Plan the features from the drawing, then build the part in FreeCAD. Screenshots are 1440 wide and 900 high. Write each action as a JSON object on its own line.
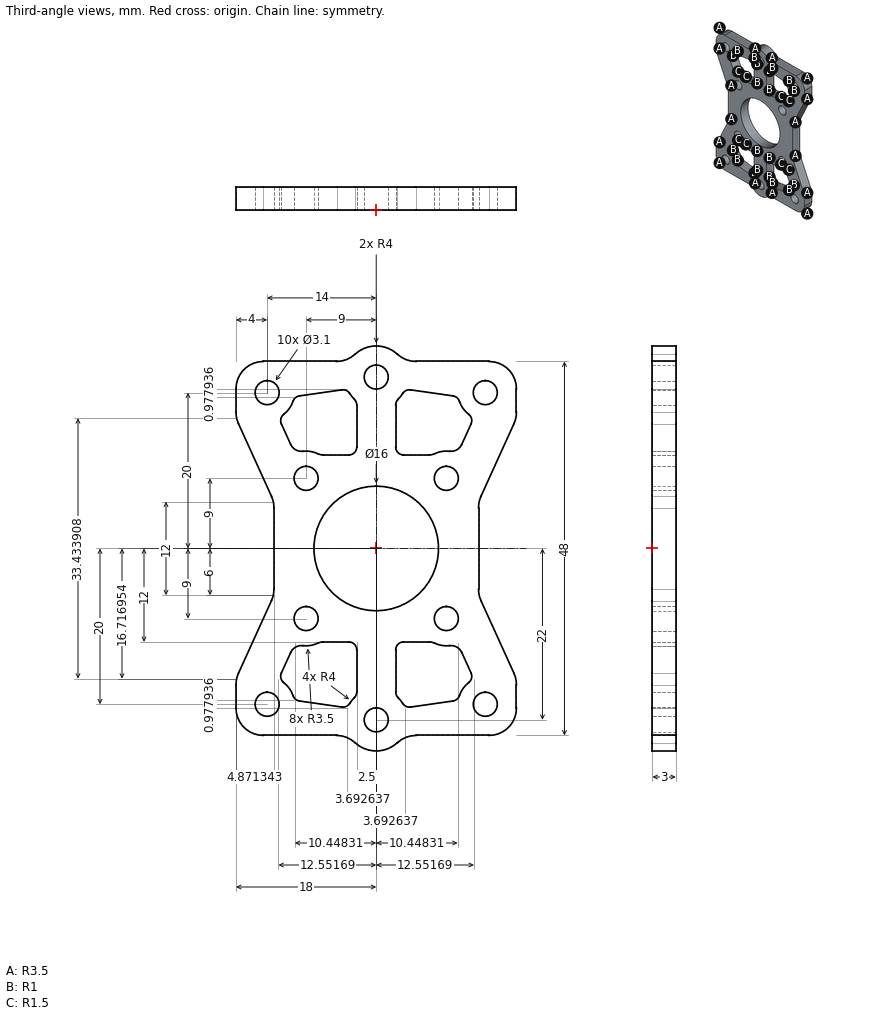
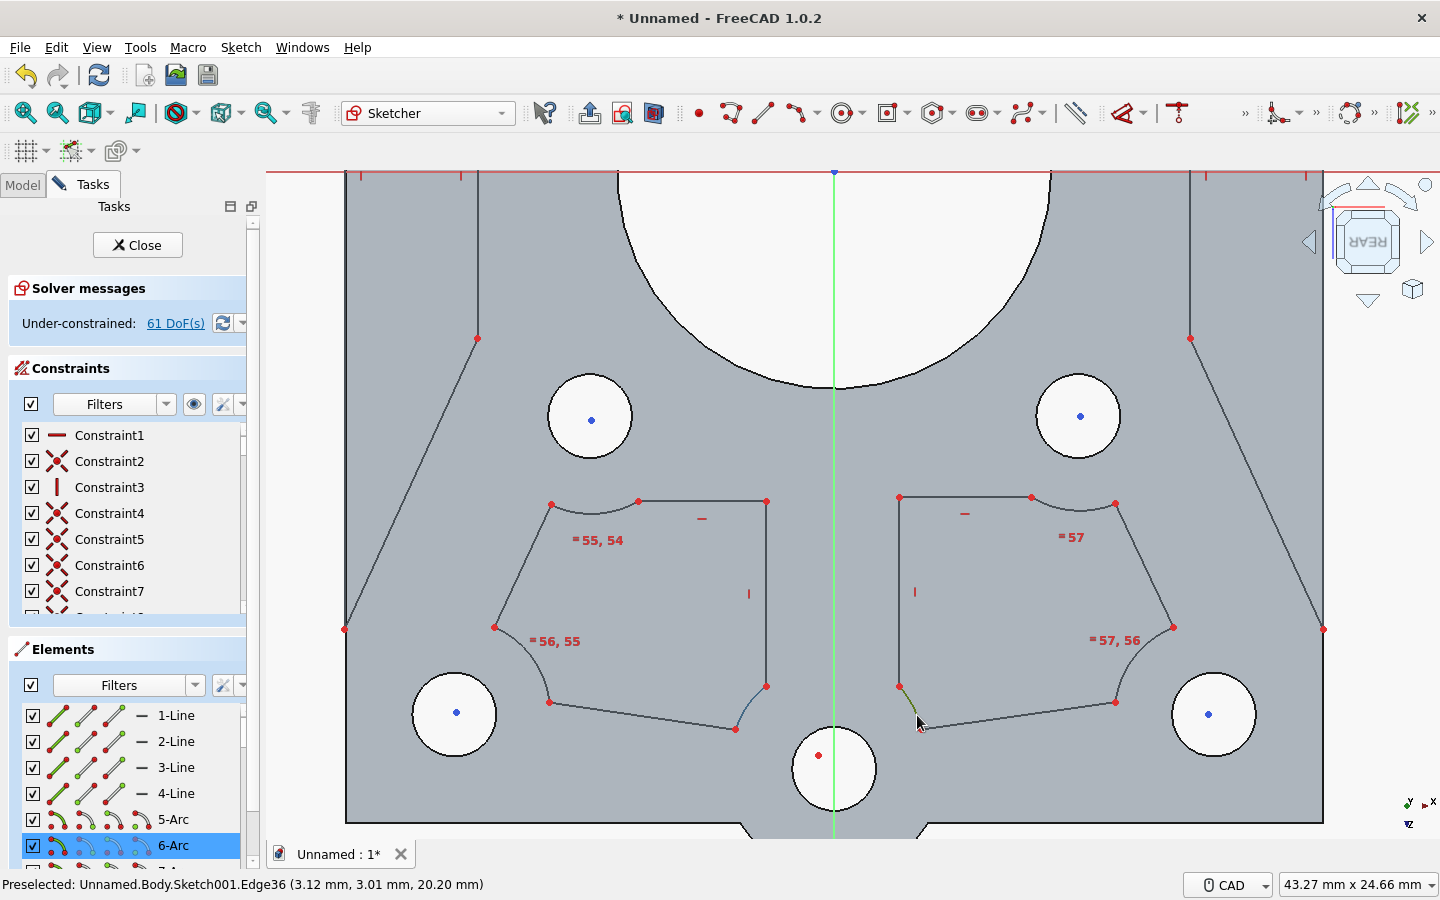
{"action": "key", "text": "e"}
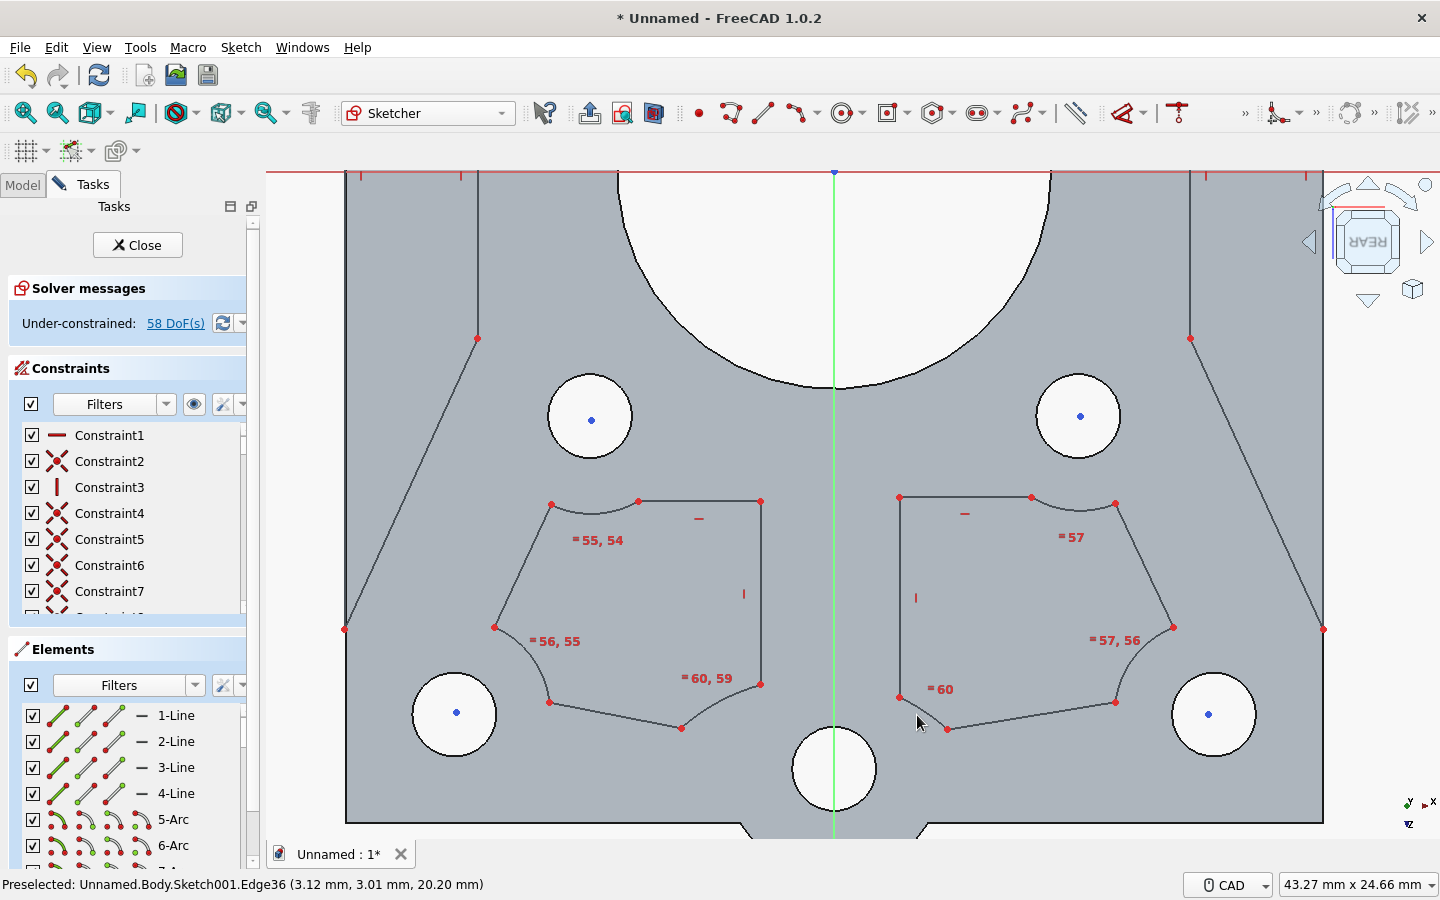
{"action": "scroll", "coordinate": [756, 698], "scroll_direction": "down", "scroll_amount": 5}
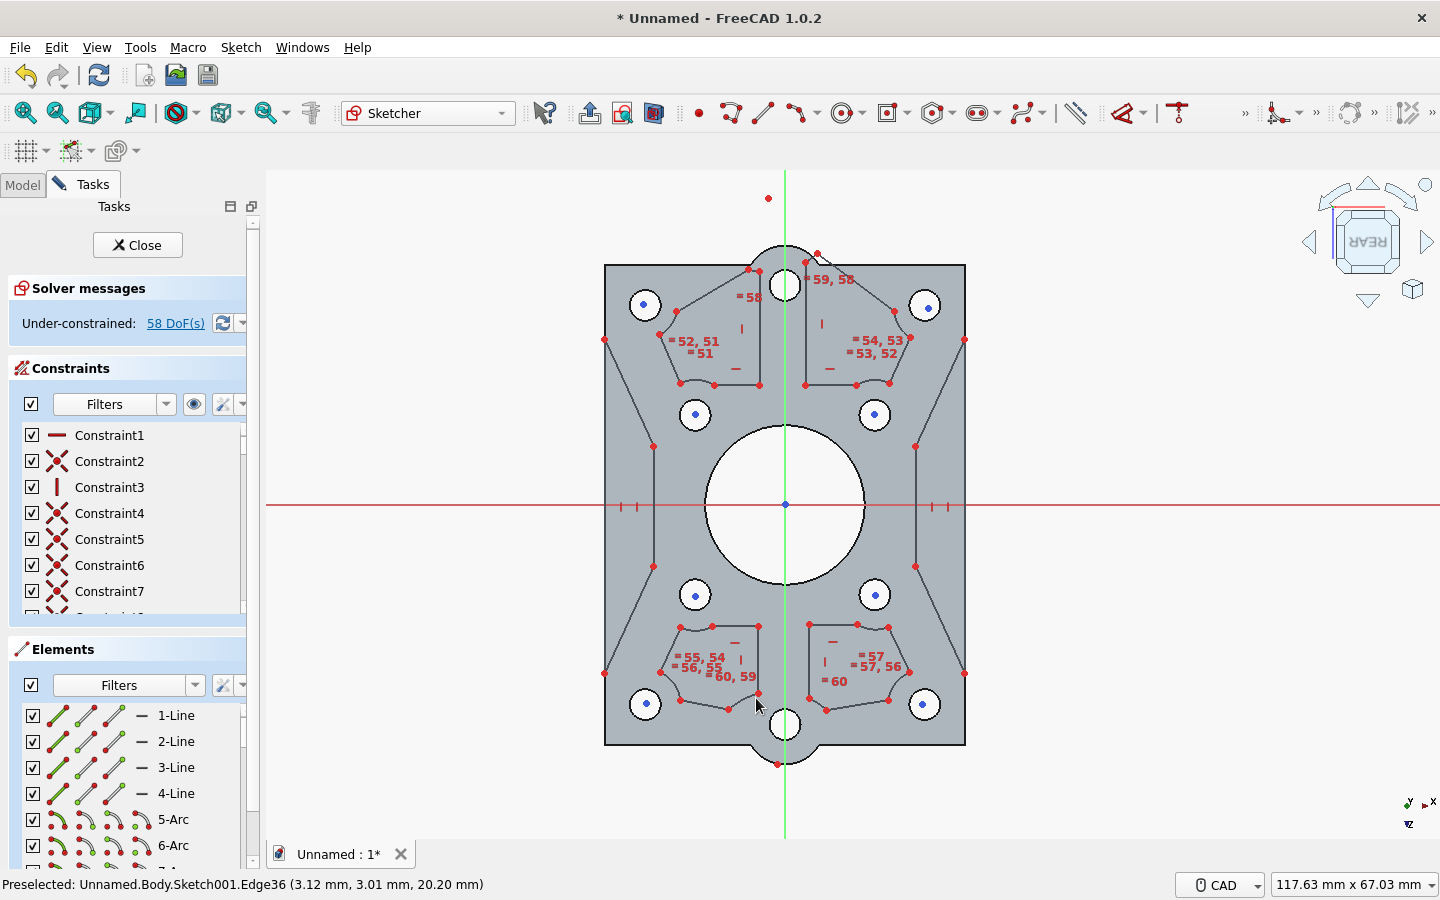
{"action": "left_click", "coordinate": [768, 199]}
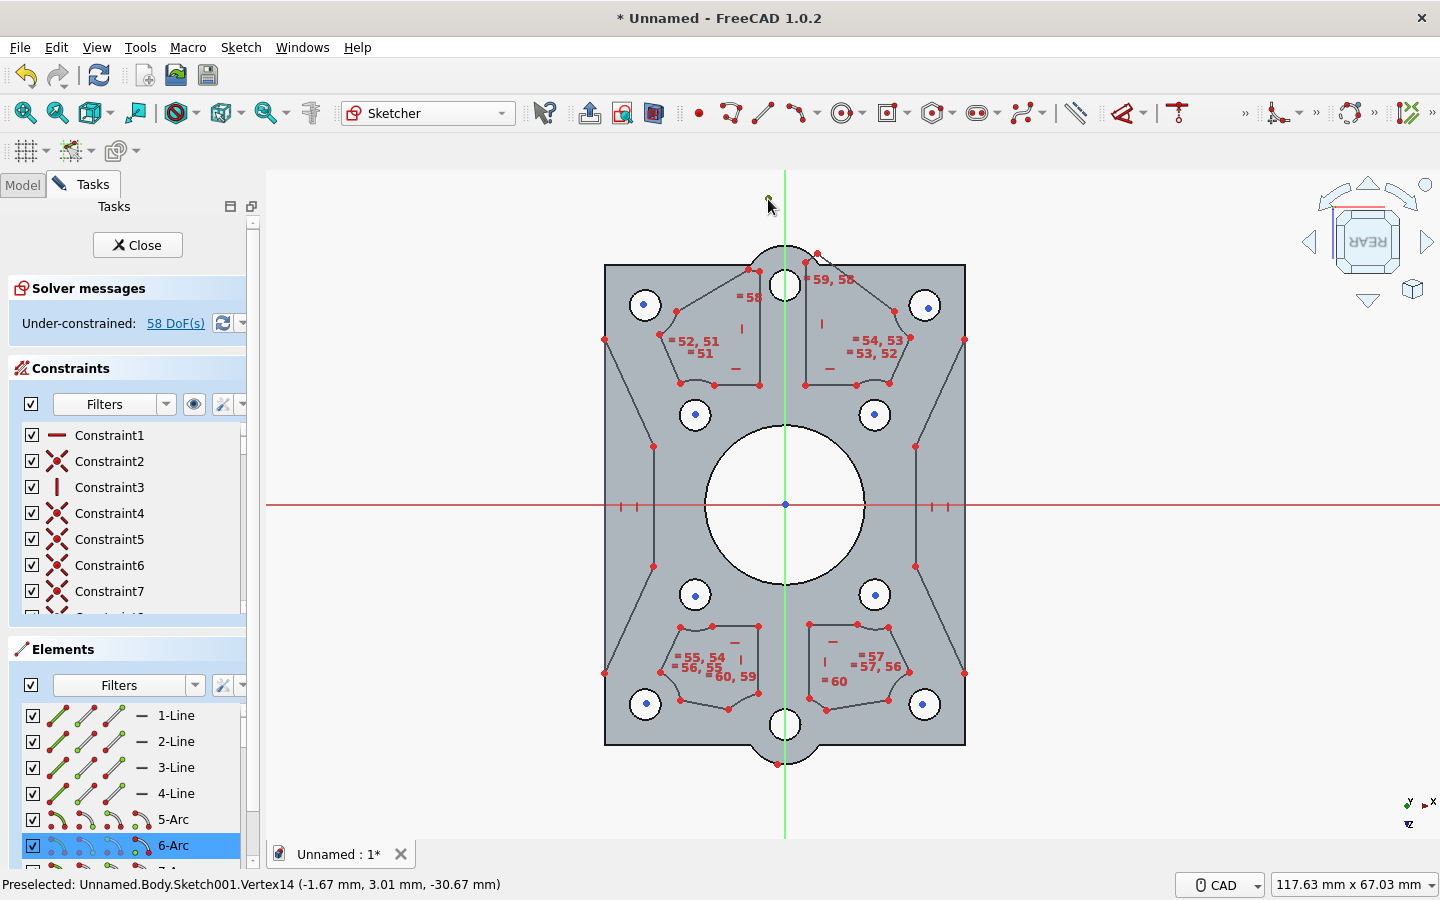
{"action": "left_click", "coordinate": [785, 767]}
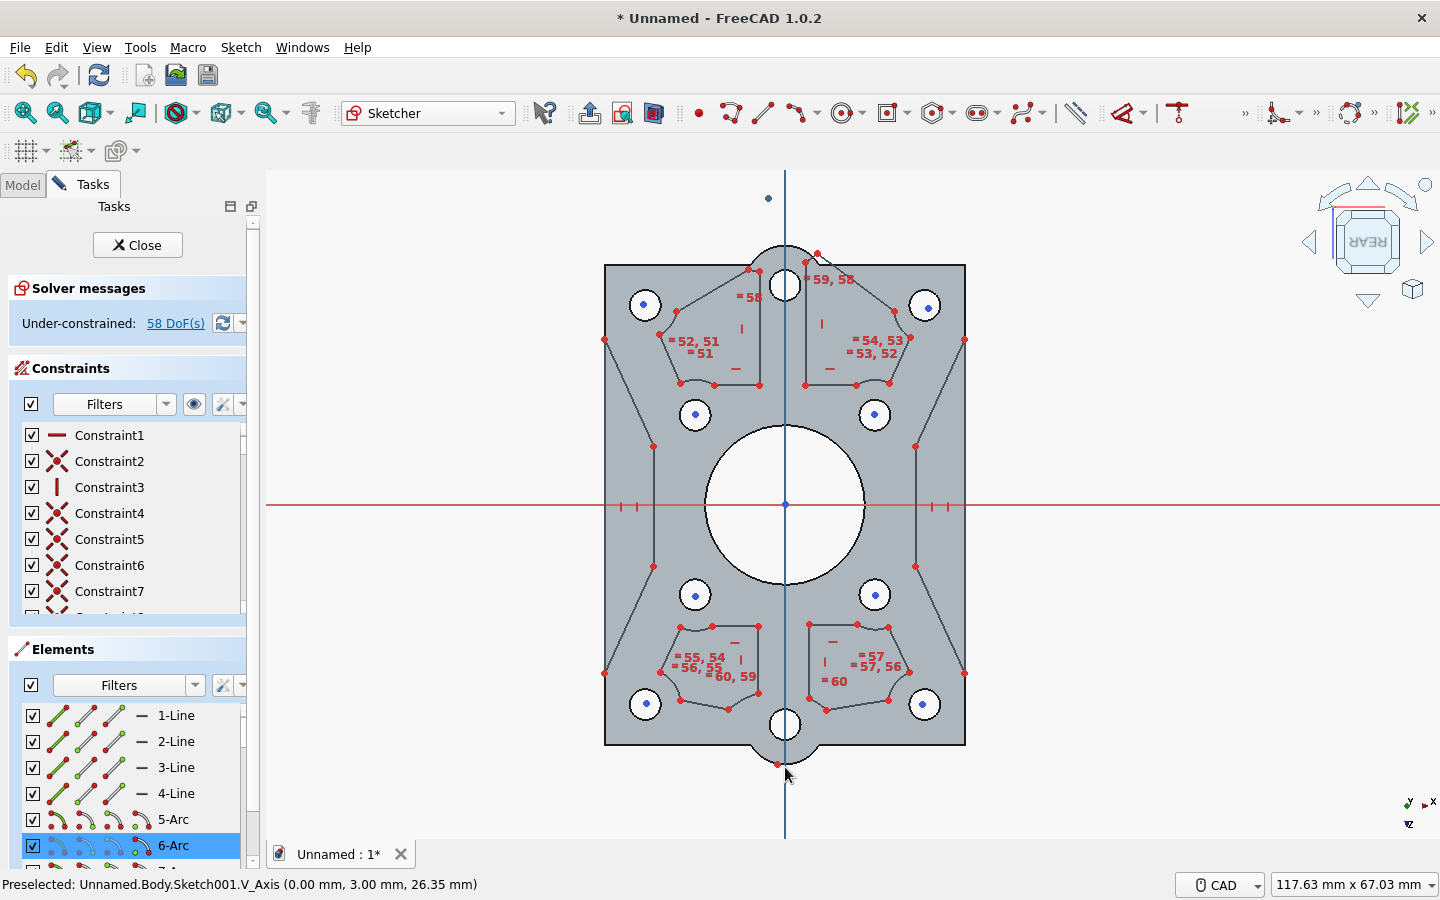
{"action": "key", "text": "c"}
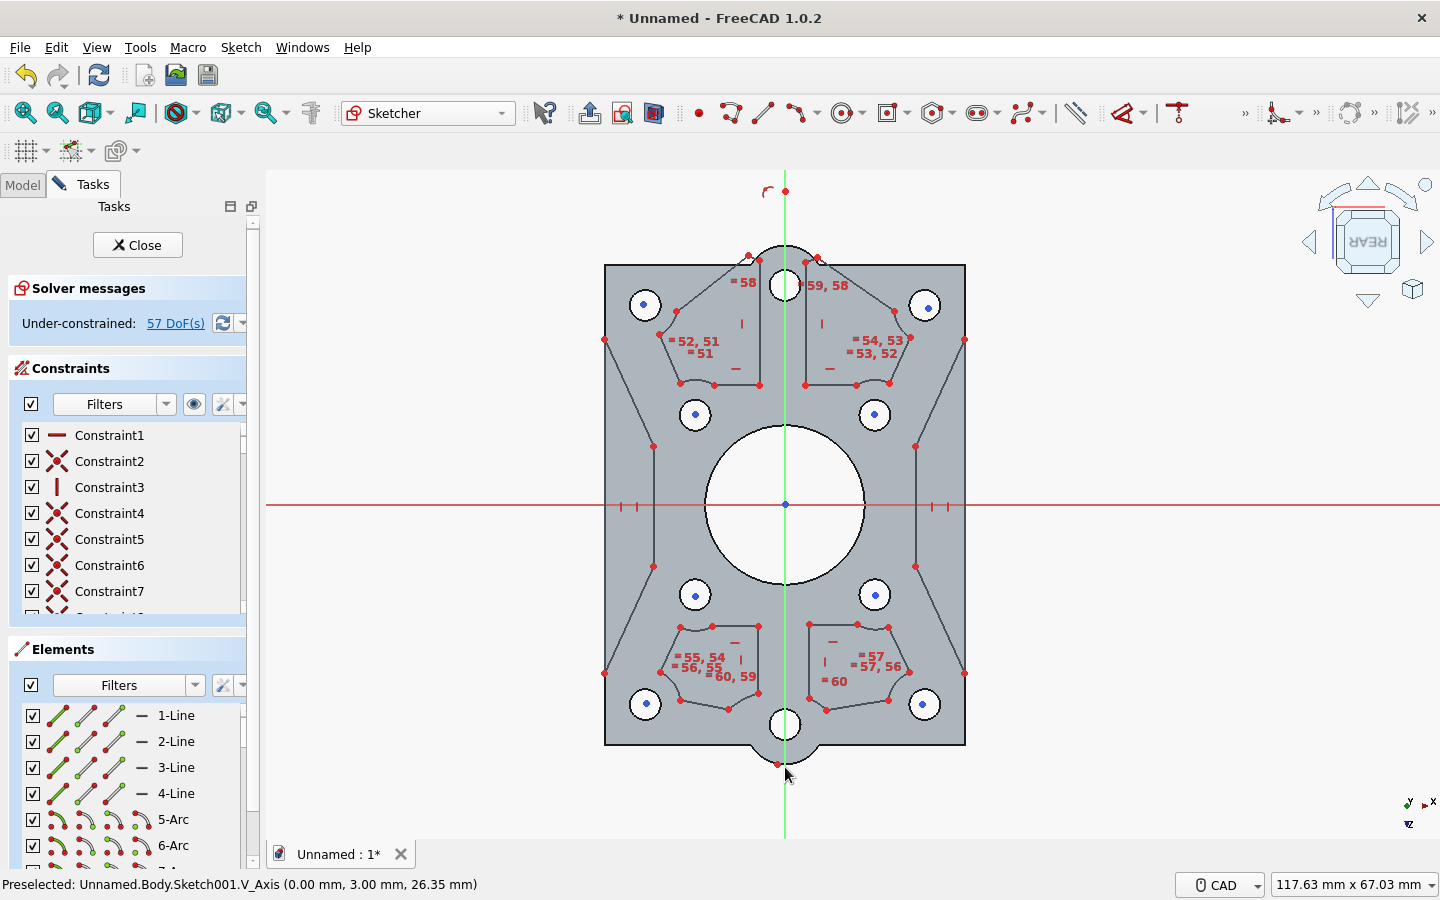
{"action": "left_click", "coordinate": [777, 765]}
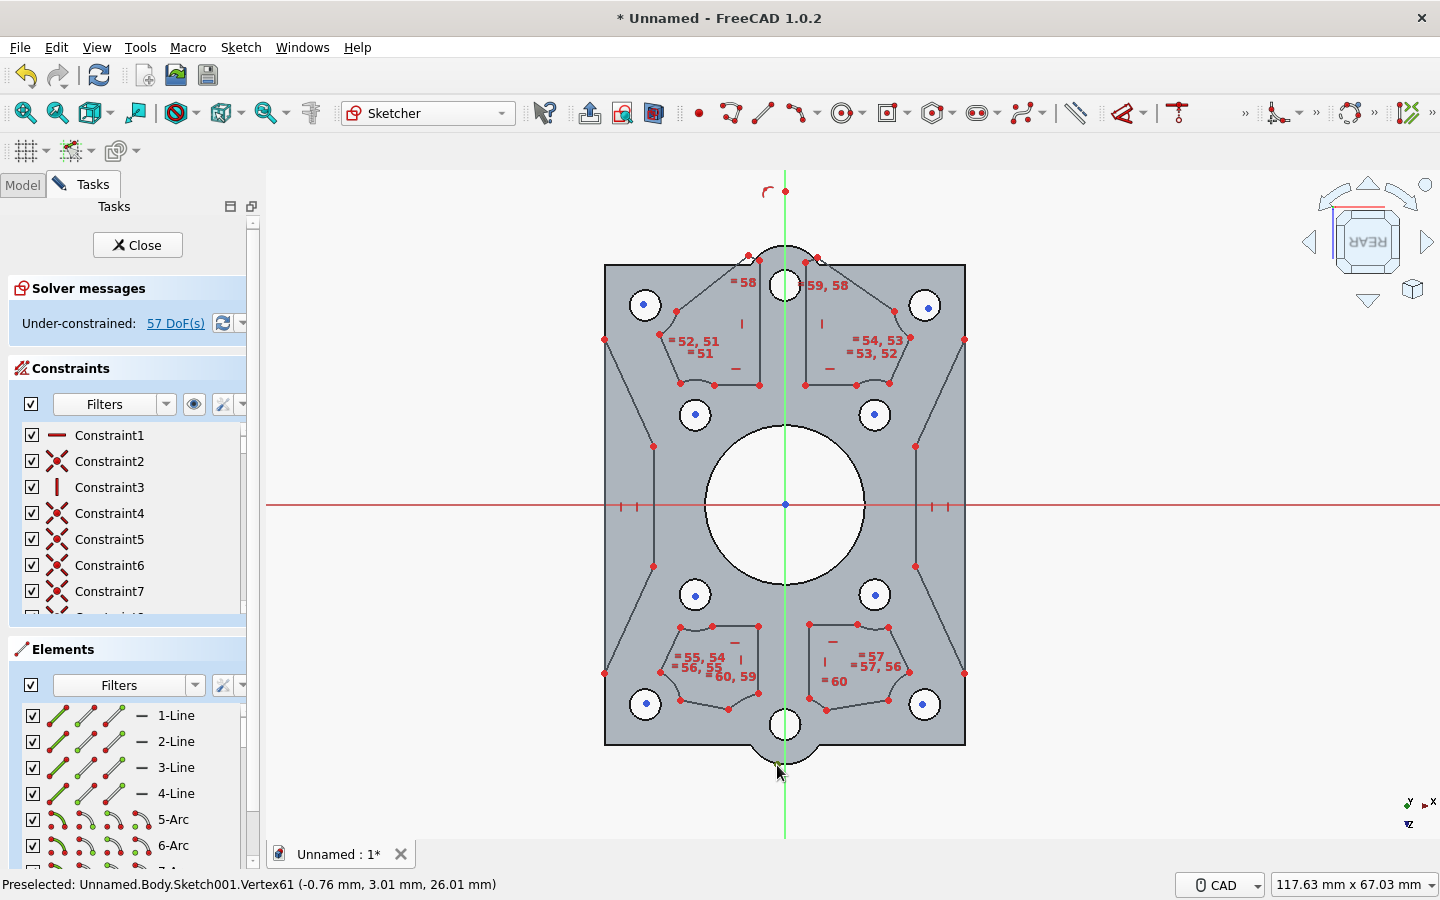
{"action": "left_click", "coordinate": [785, 767]}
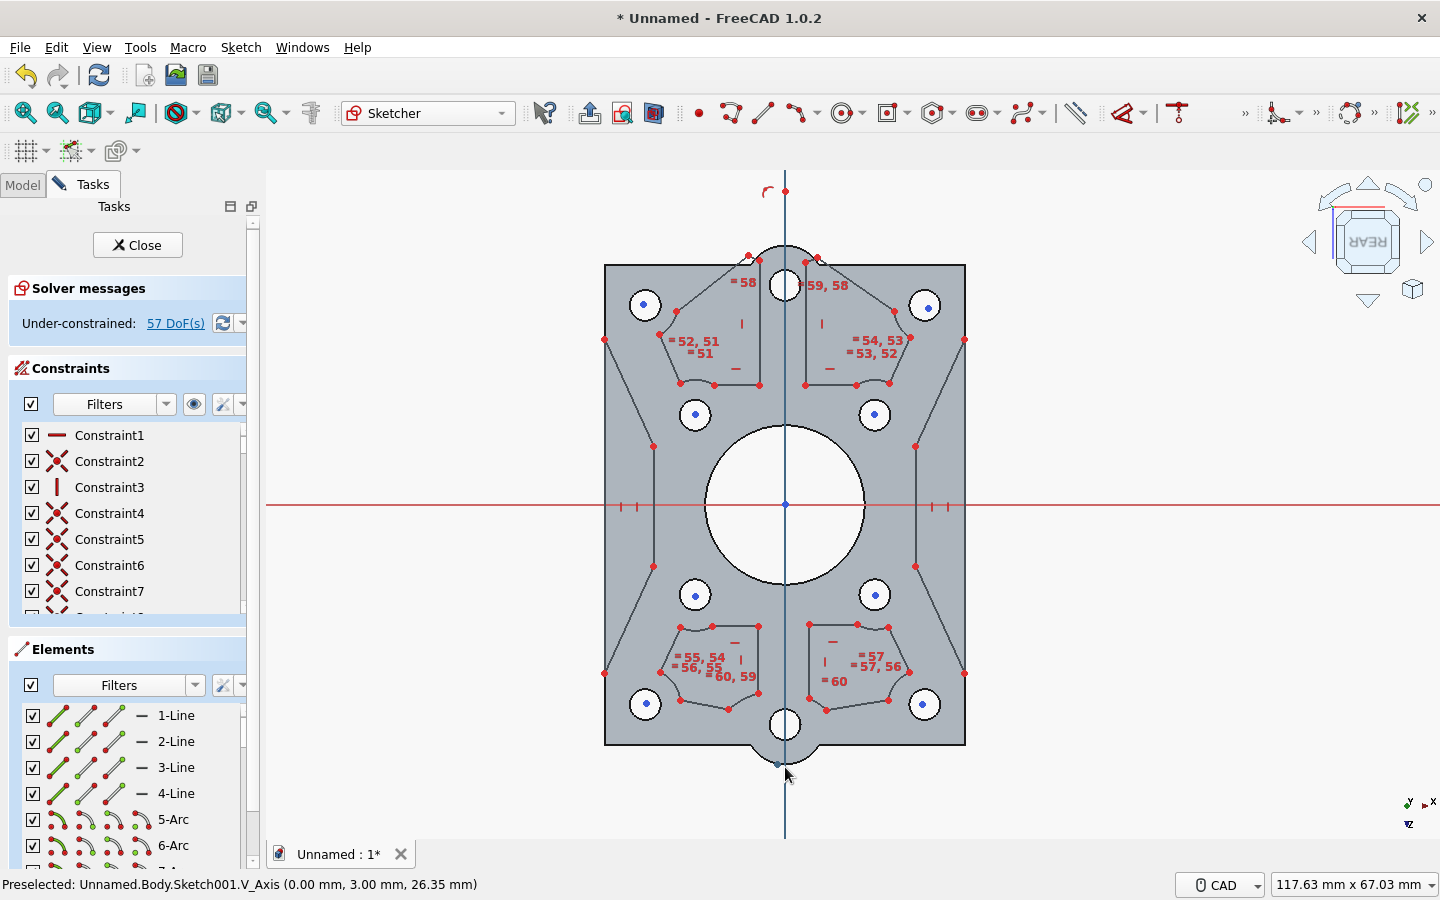
{"action": "key", "text": "c"}